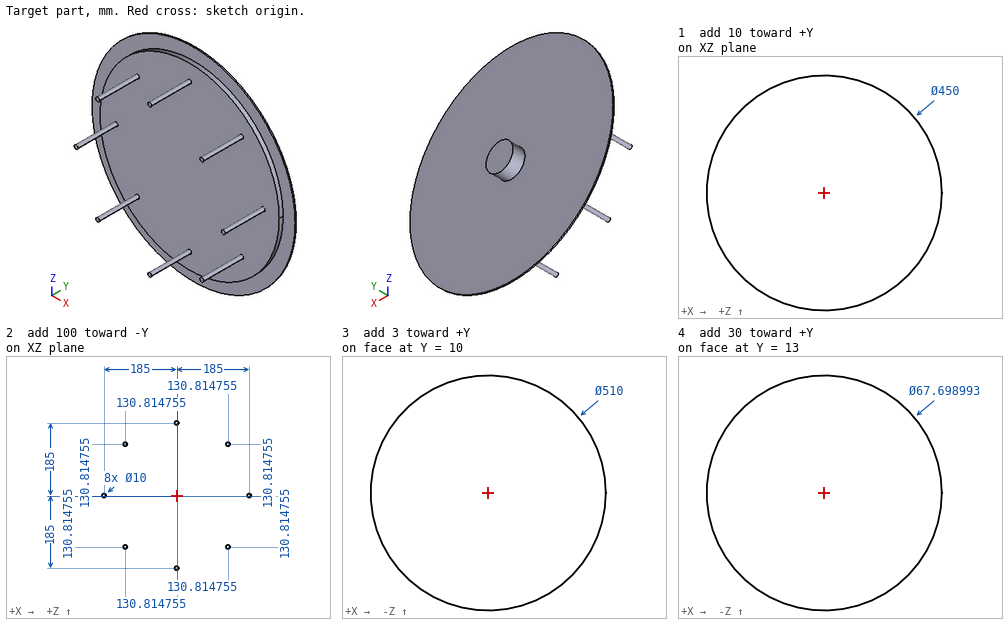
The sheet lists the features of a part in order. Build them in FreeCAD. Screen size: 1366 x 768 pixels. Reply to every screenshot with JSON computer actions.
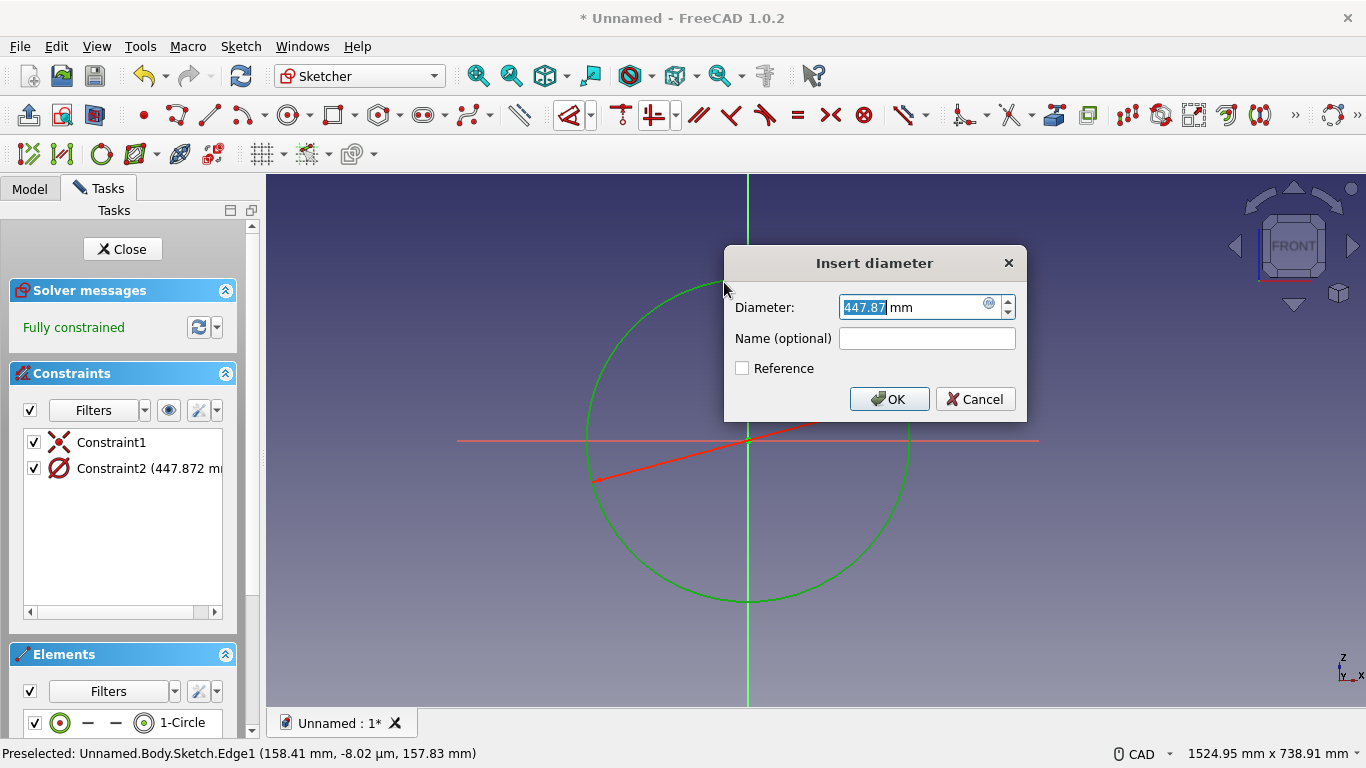
{"action": "type", "text": "450"}
{"action": "key", "text": "Return"}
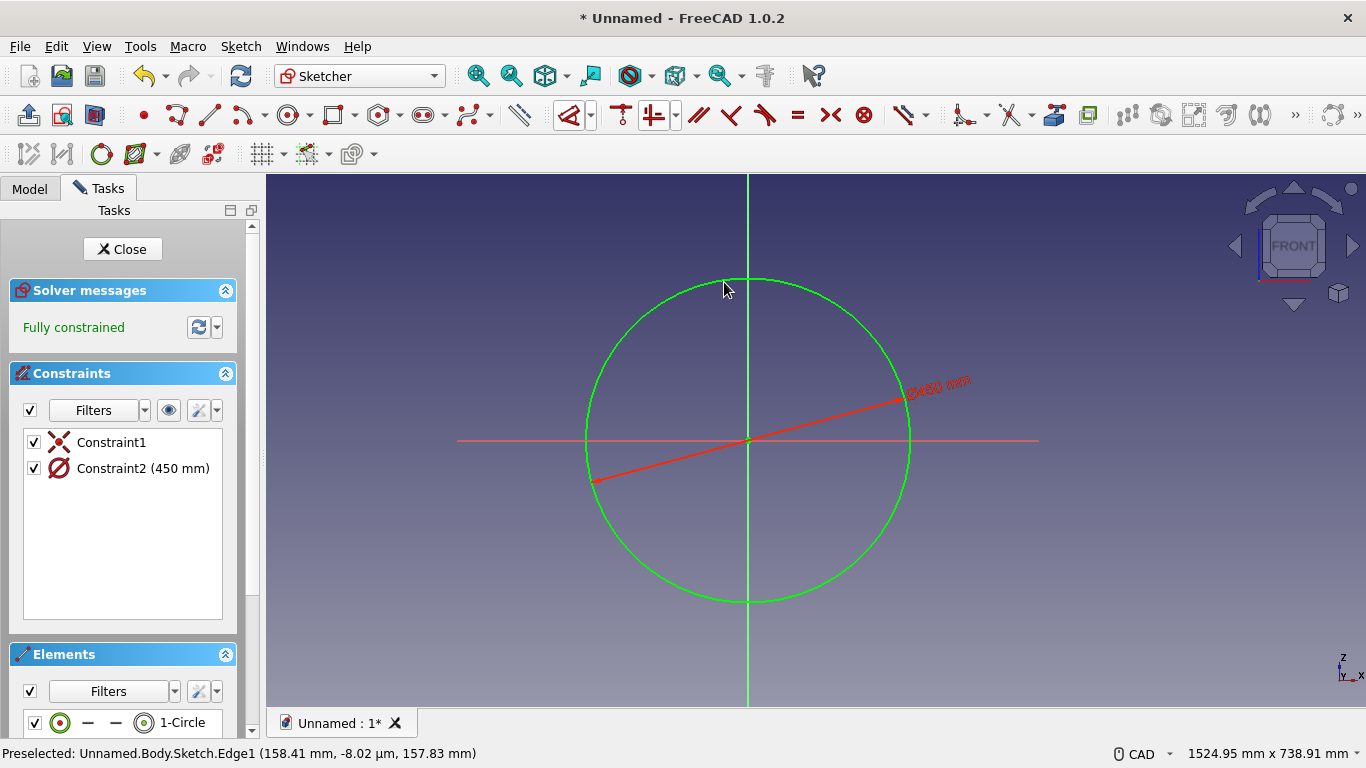
{"action": "left_click", "coordinate": [123, 249]}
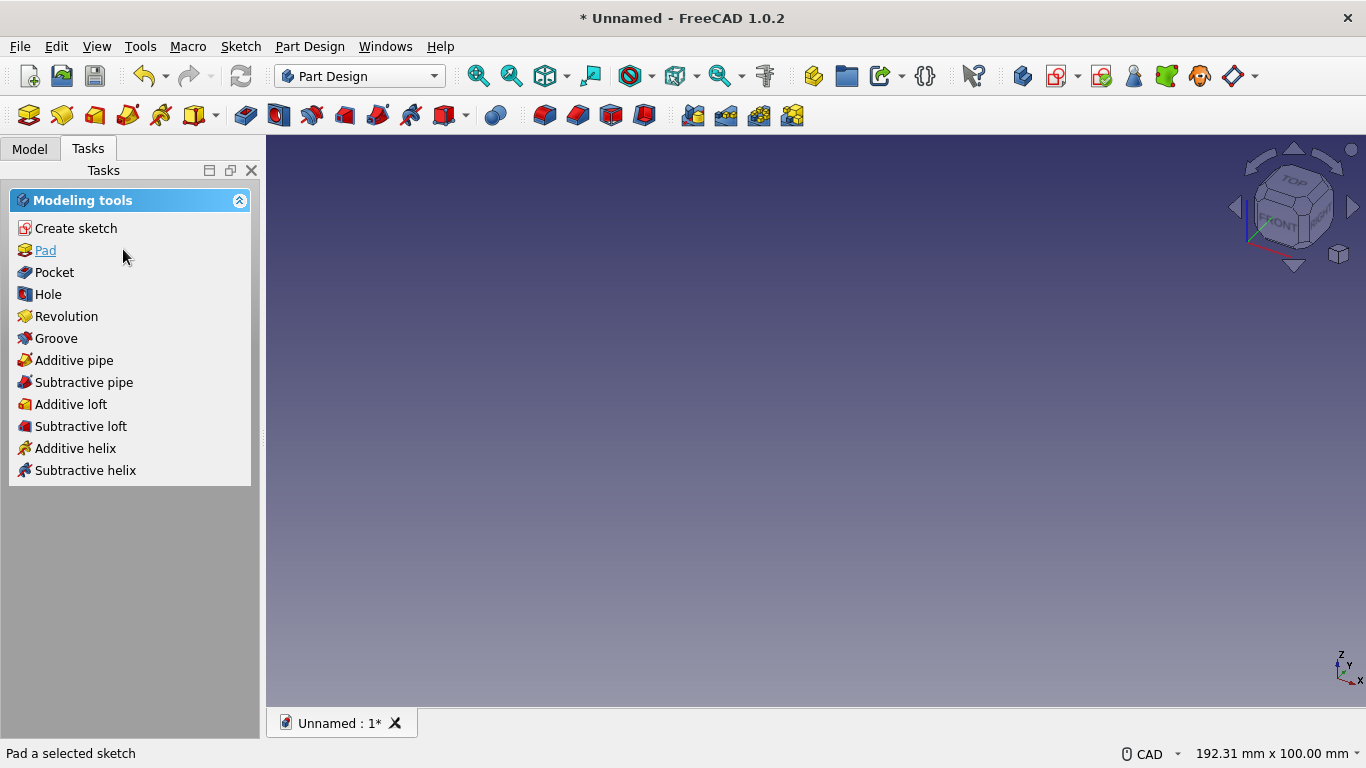
{"action": "left_click", "coordinate": [29, 116]}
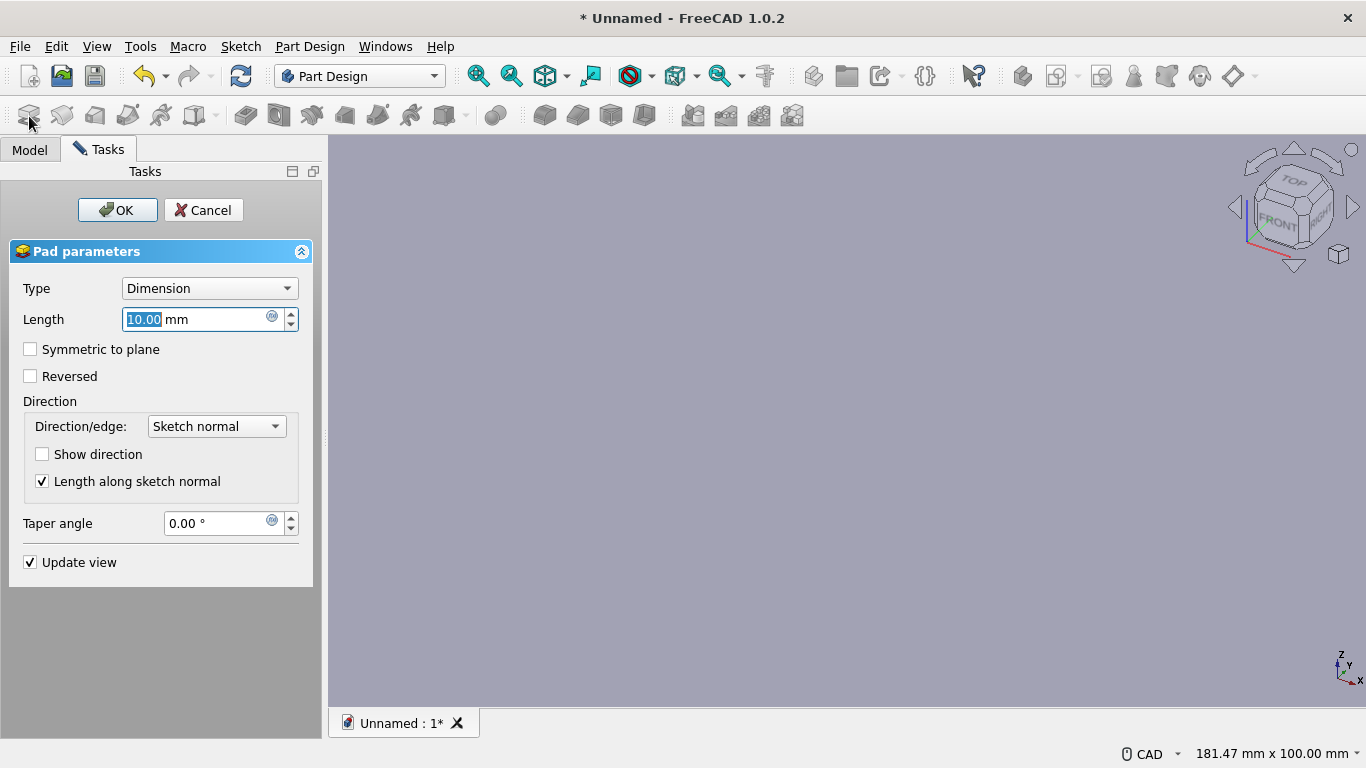
{"action": "type", "text": "10"}
{"action": "key", "text": "Tab"}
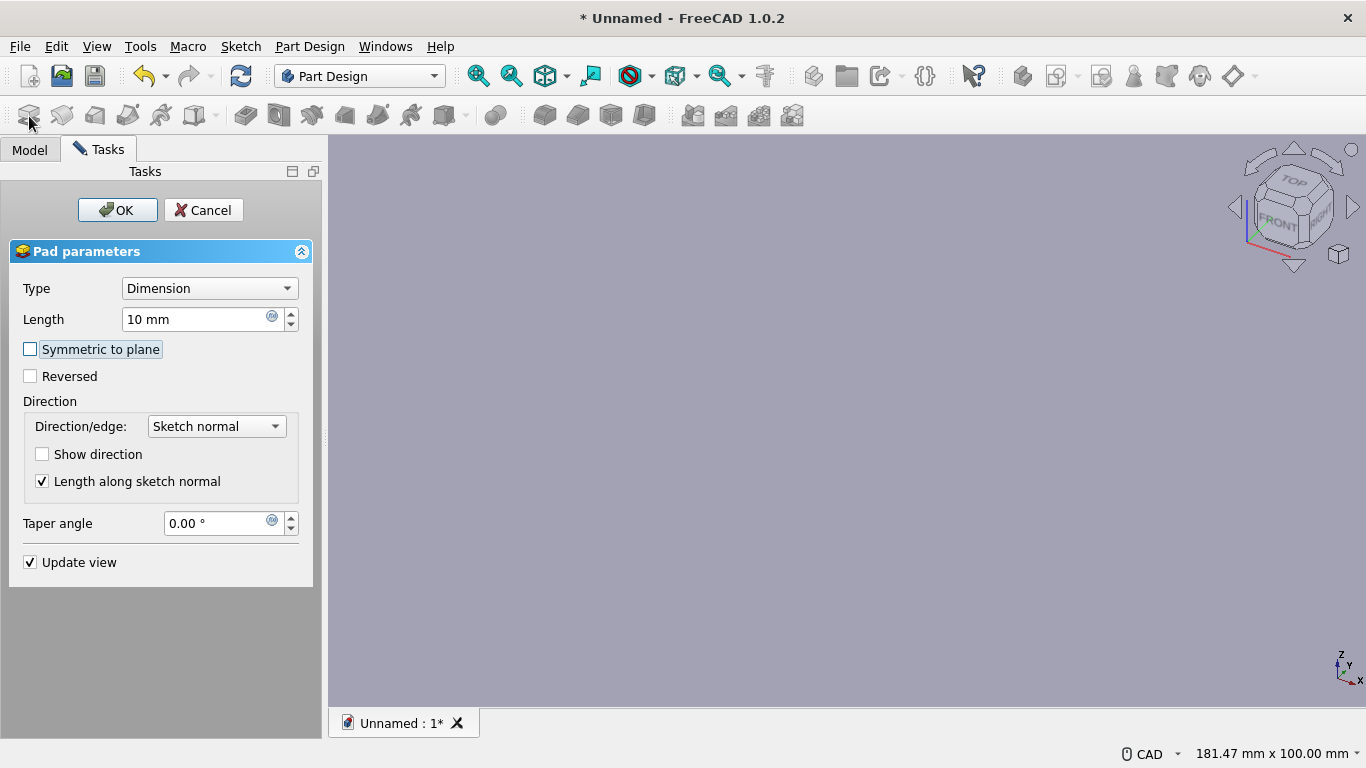
{"action": "left_click", "coordinate": [31, 376]}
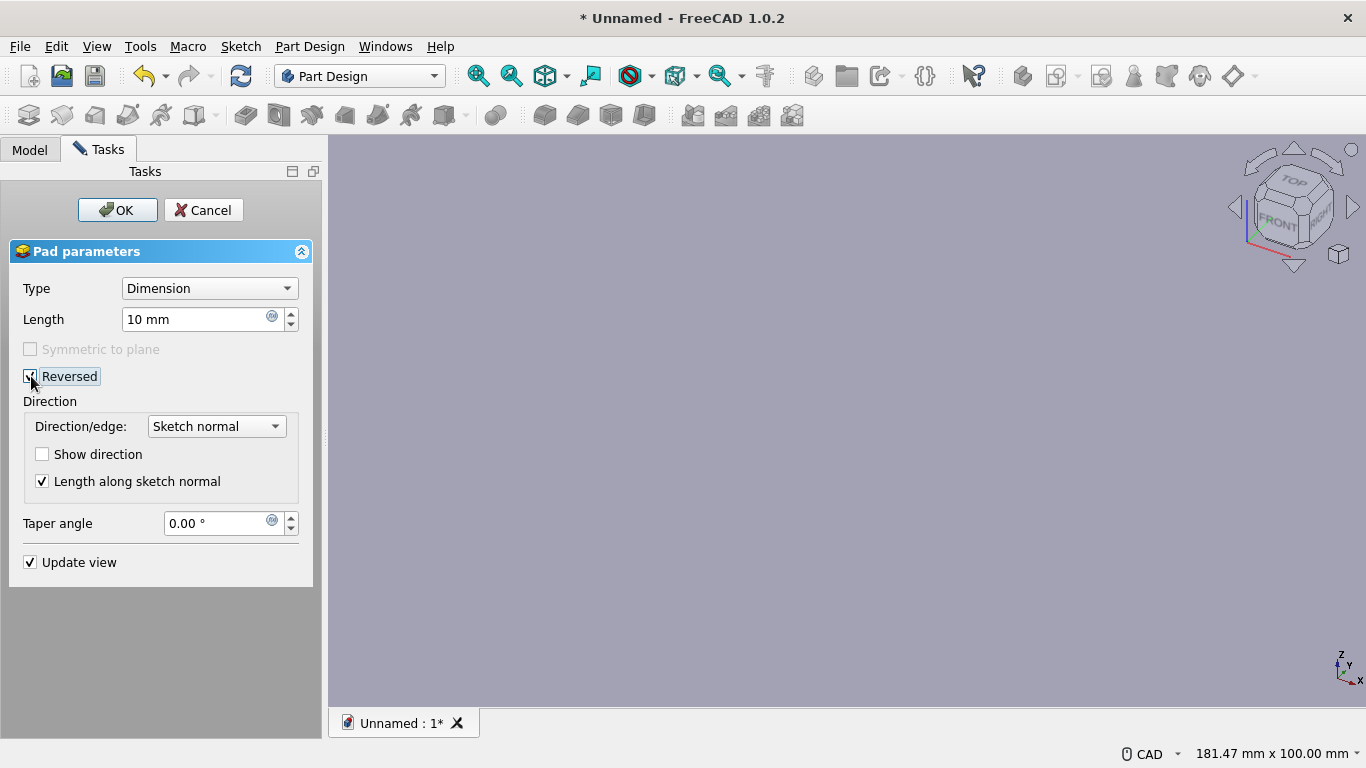
{"action": "left_click", "coordinate": [118, 210]}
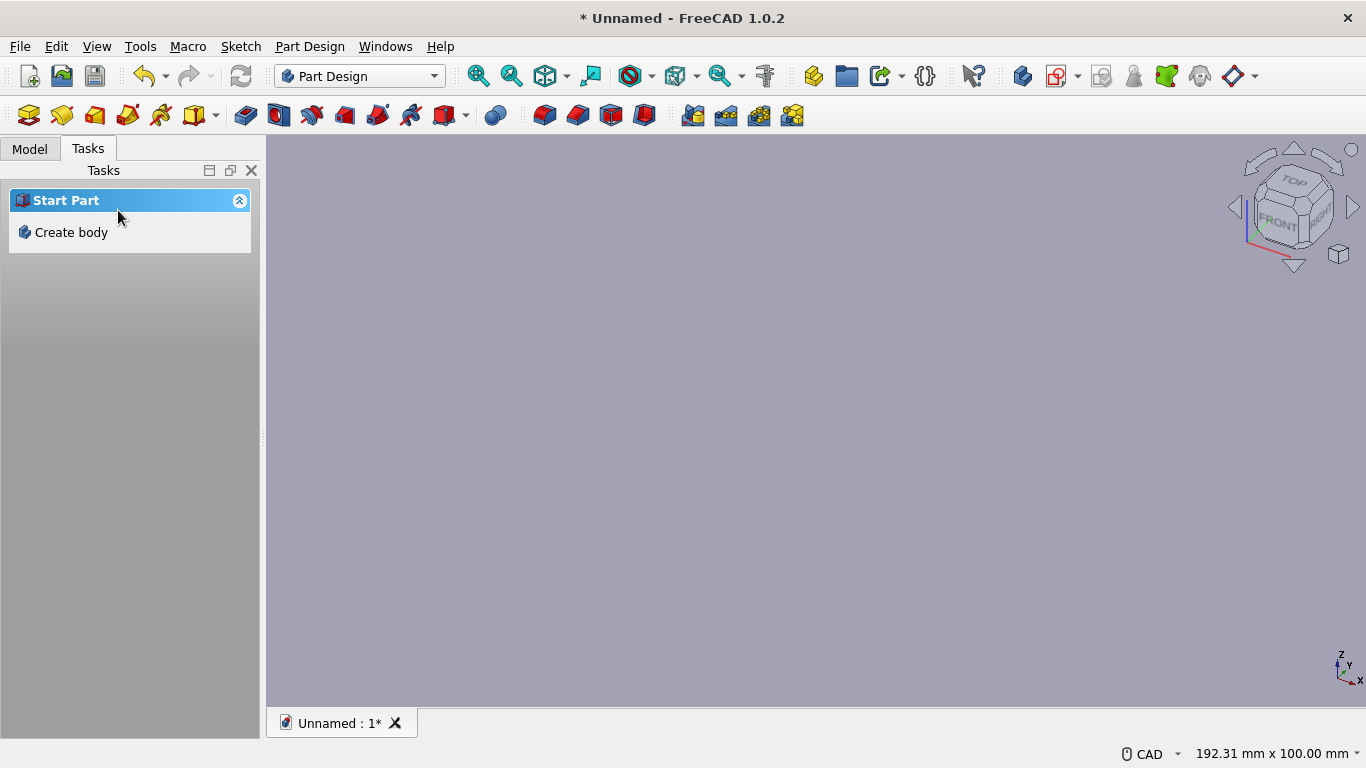
{"action": "left_click", "coordinate": [479, 76]}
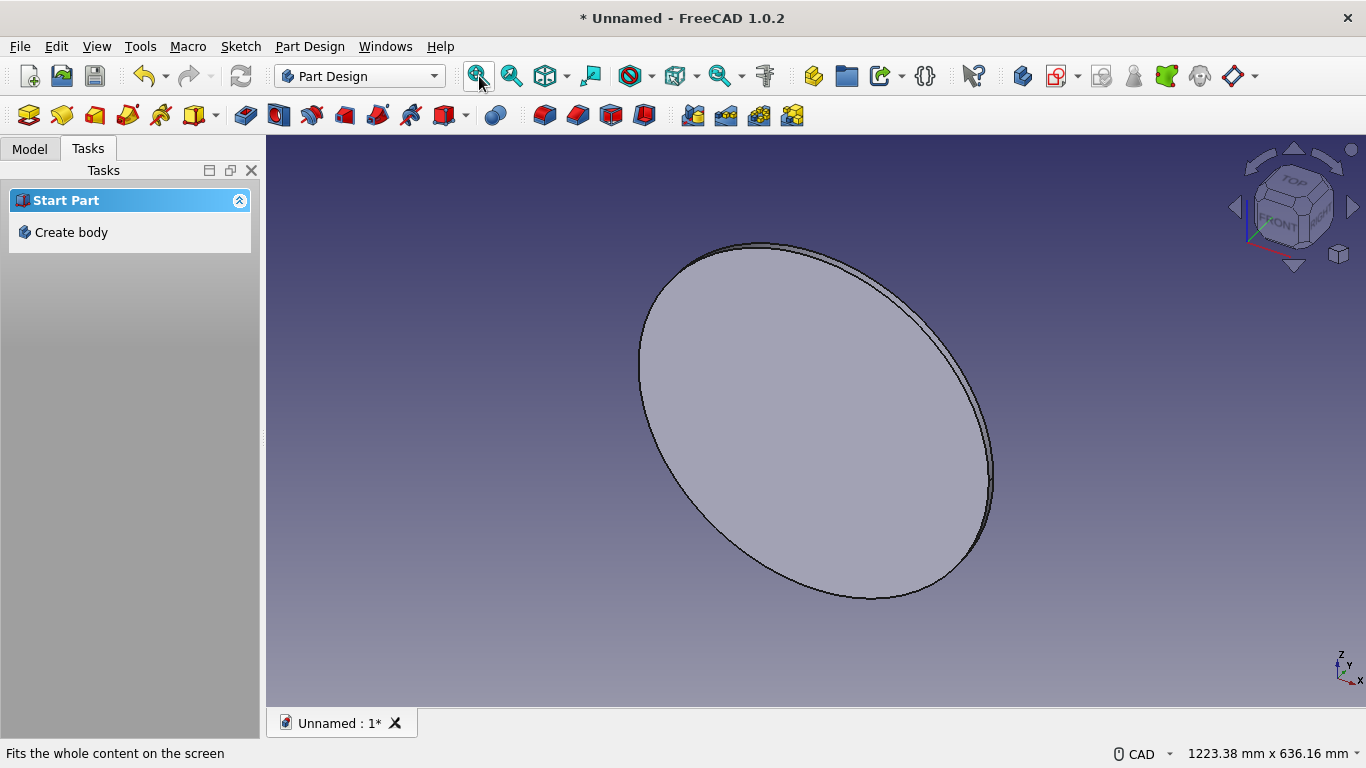
{"action": "left_click", "coordinate": [1056, 76]}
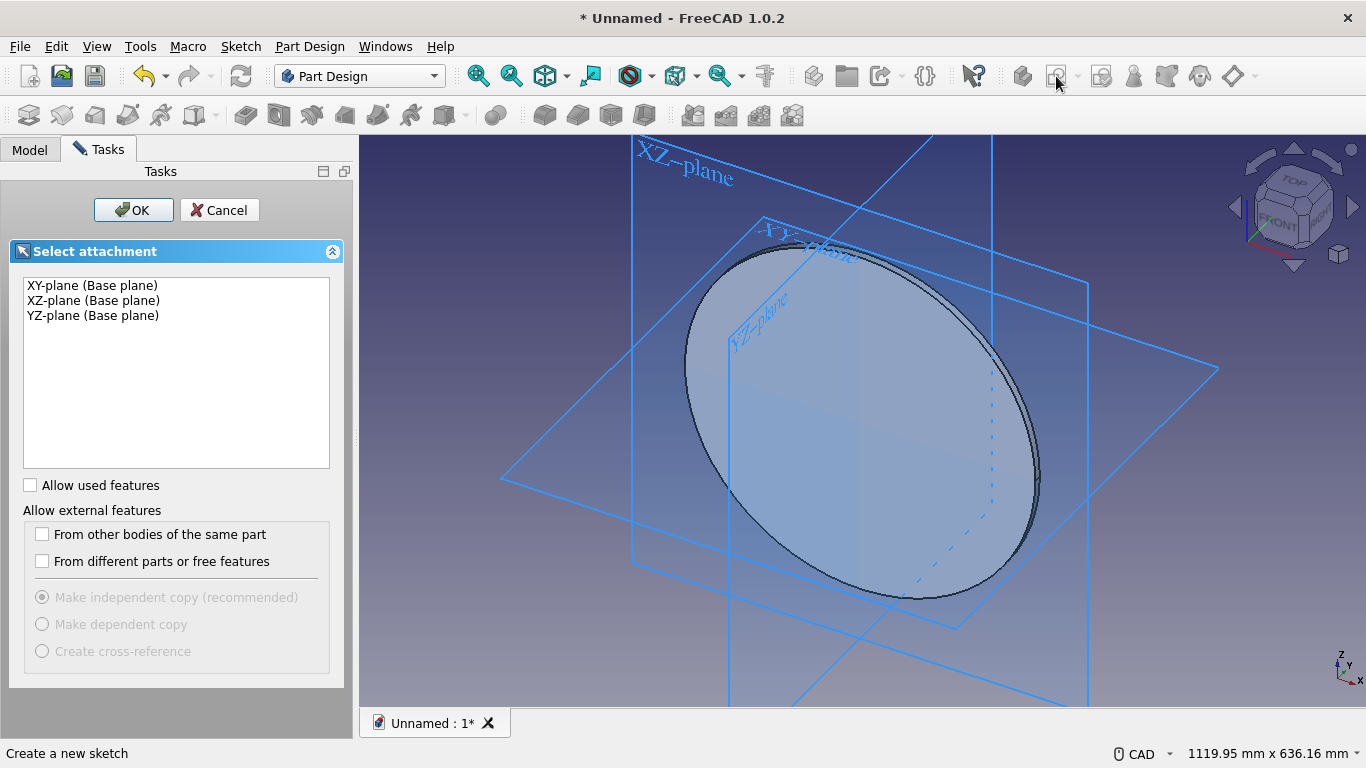
{"action": "left_click", "coordinate": [84, 300]}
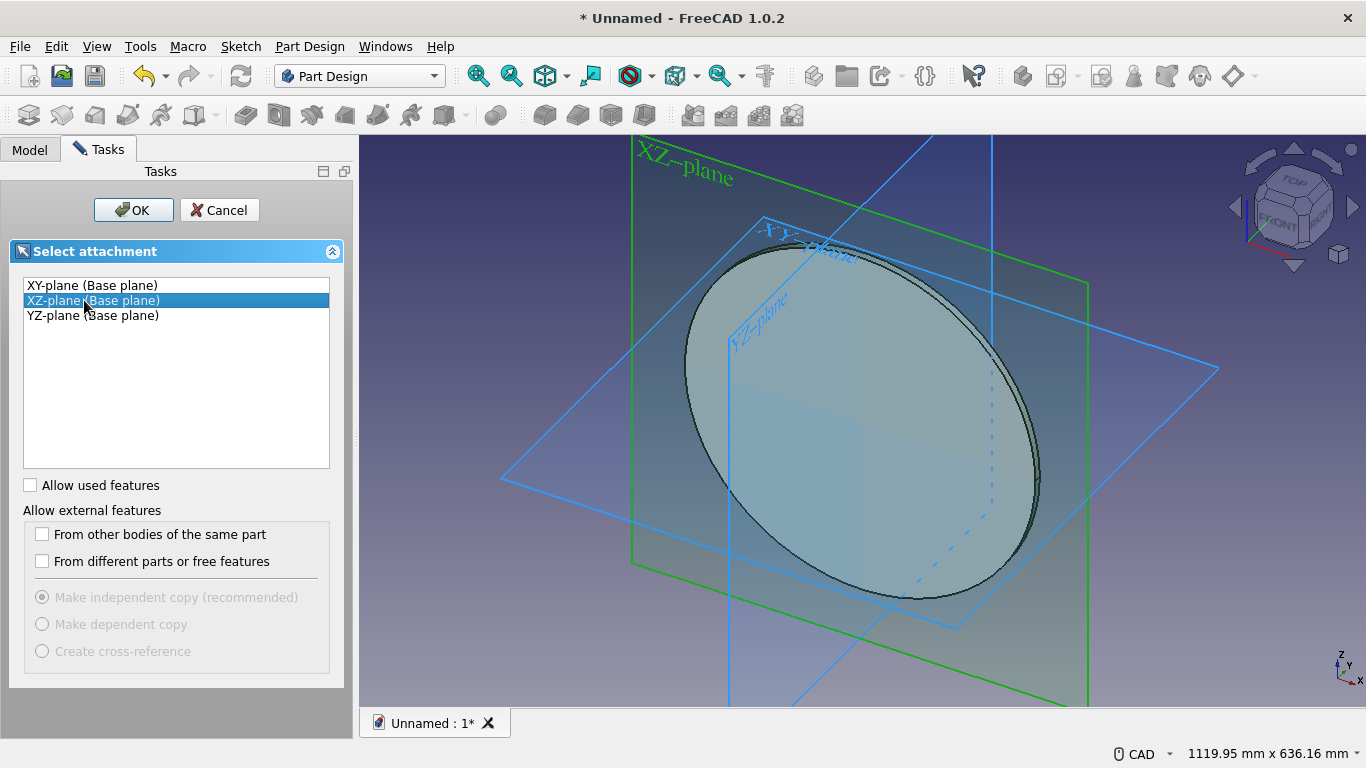
{"action": "left_click", "coordinate": [134, 210]}